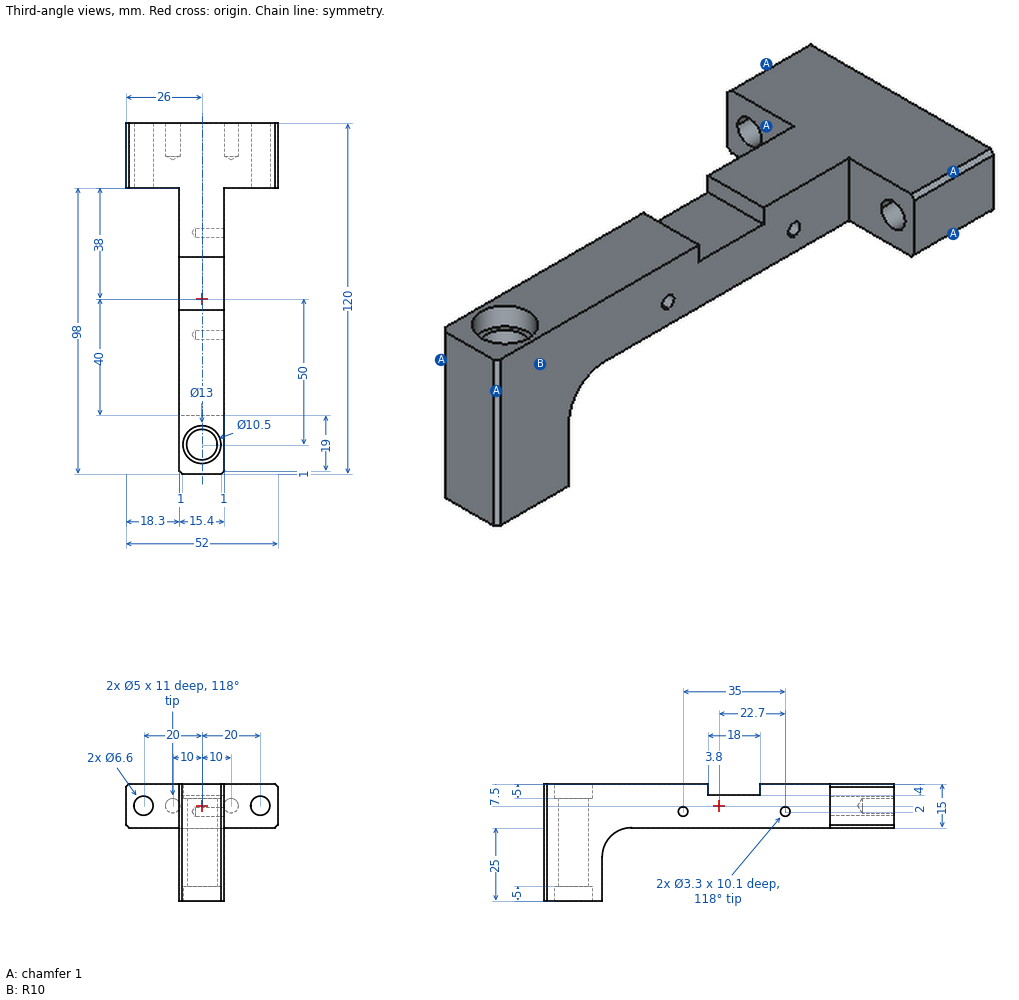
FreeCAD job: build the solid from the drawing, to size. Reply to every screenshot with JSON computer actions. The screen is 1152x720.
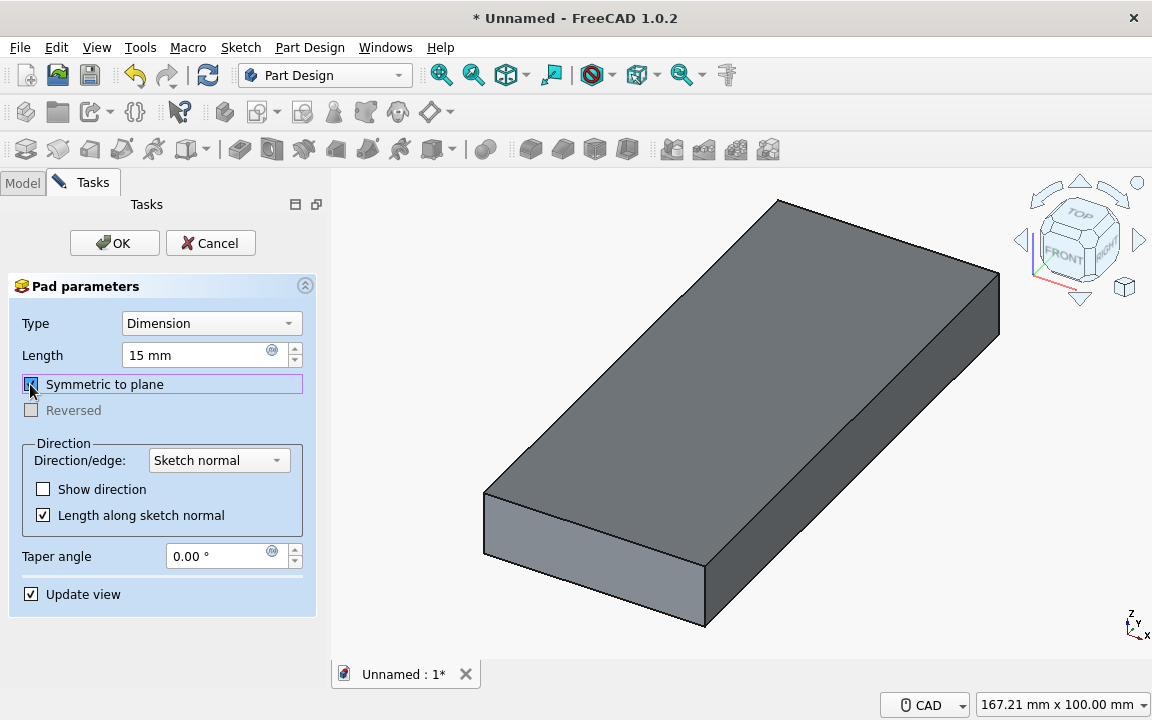
{"action": "left_click", "coordinate": [115, 243]}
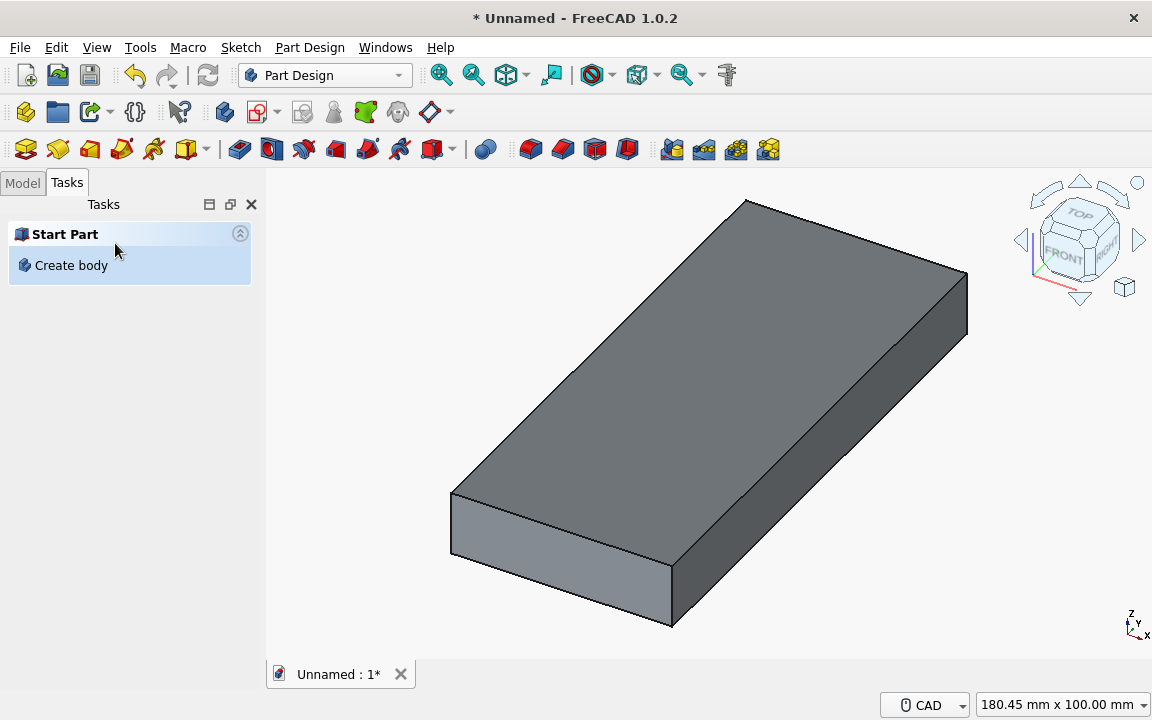
{"action": "left_click", "coordinate": [751, 341]}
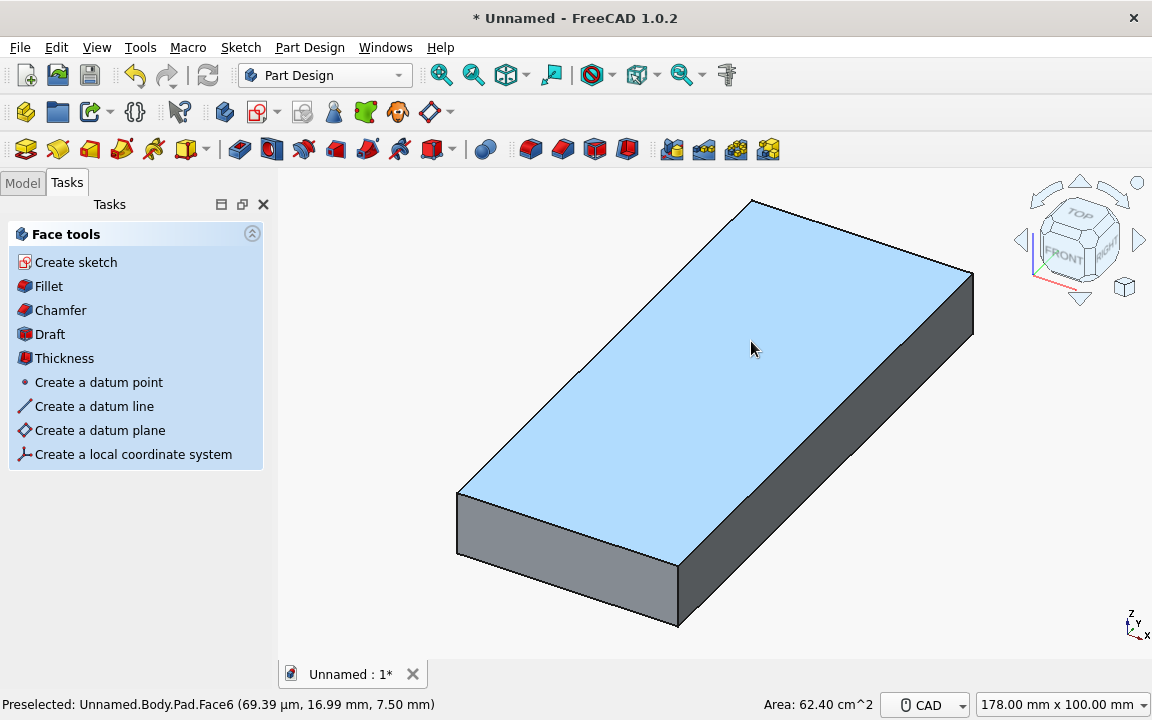
{"action": "left_click", "coordinate": [258, 112]}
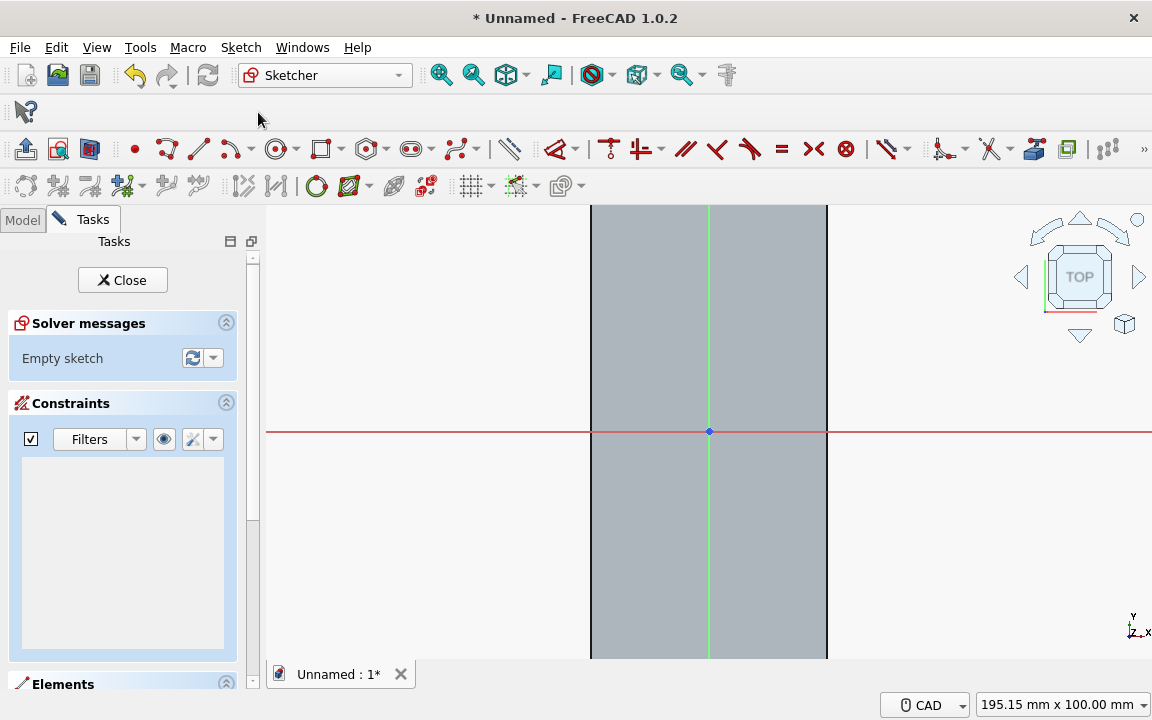
{"action": "scroll", "coordinate": [621, 330], "scroll_direction": "down", "scroll_amount": 2}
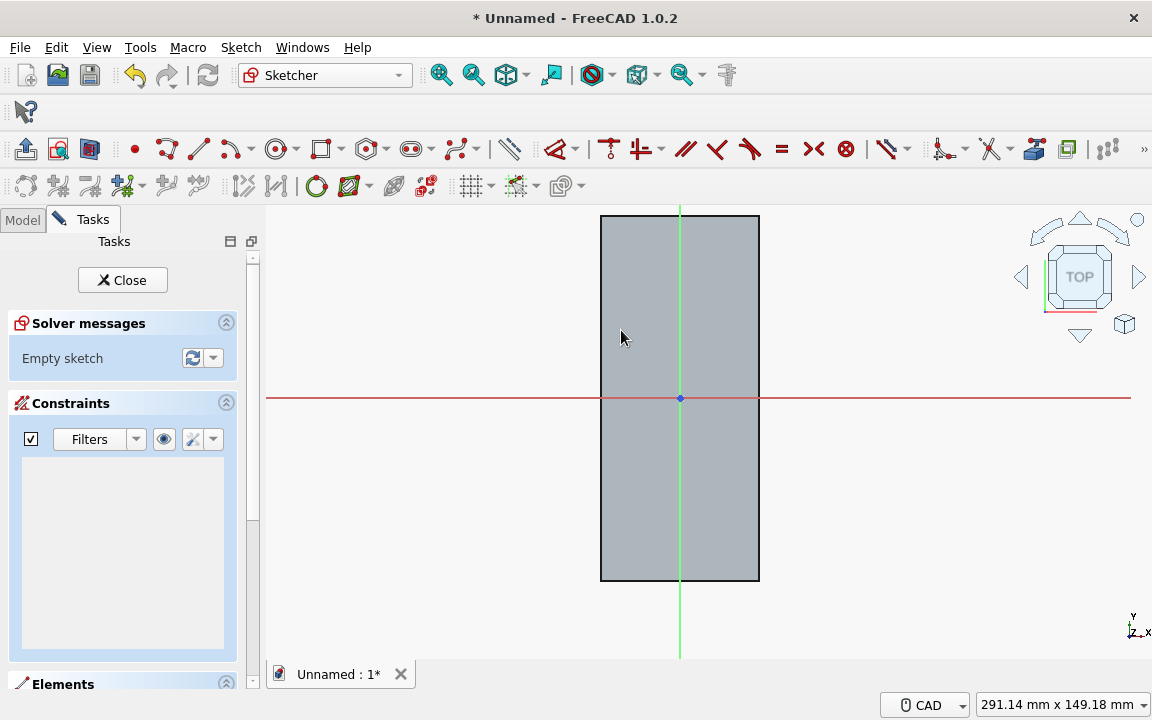
{"action": "left_click", "coordinate": [322, 150]}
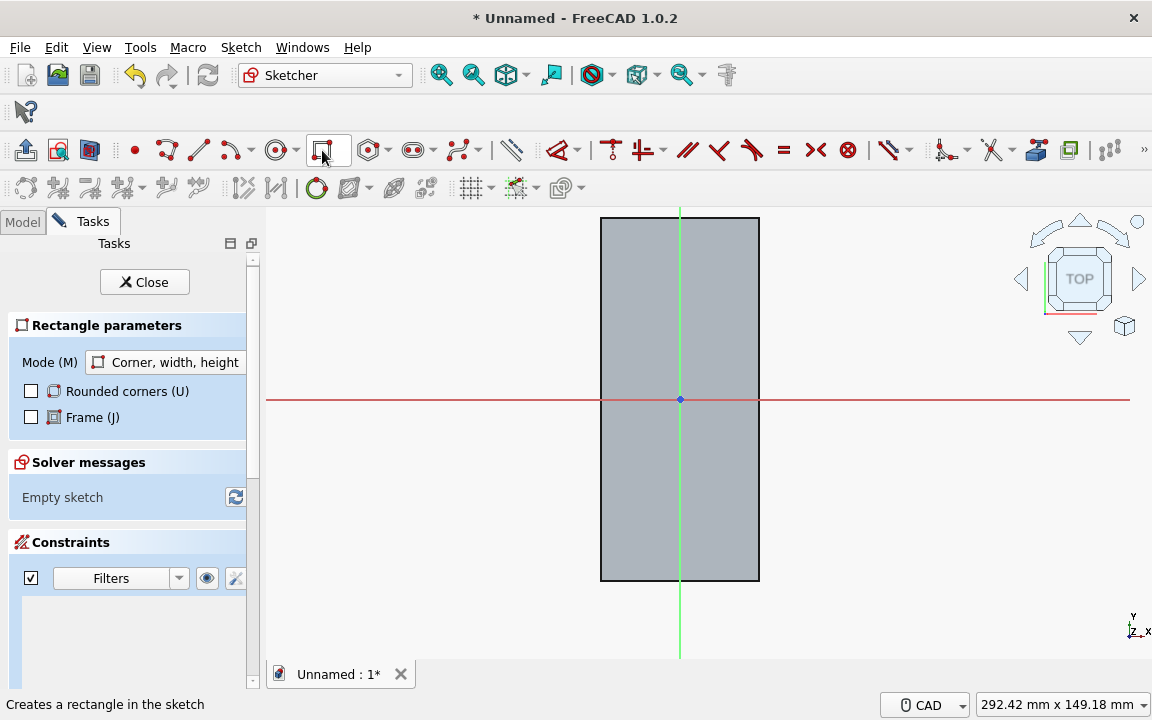
{"action": "left_click", "coordinate": [601, 284]}
{"action": "mouse_move", "coordinate": [657, 581]}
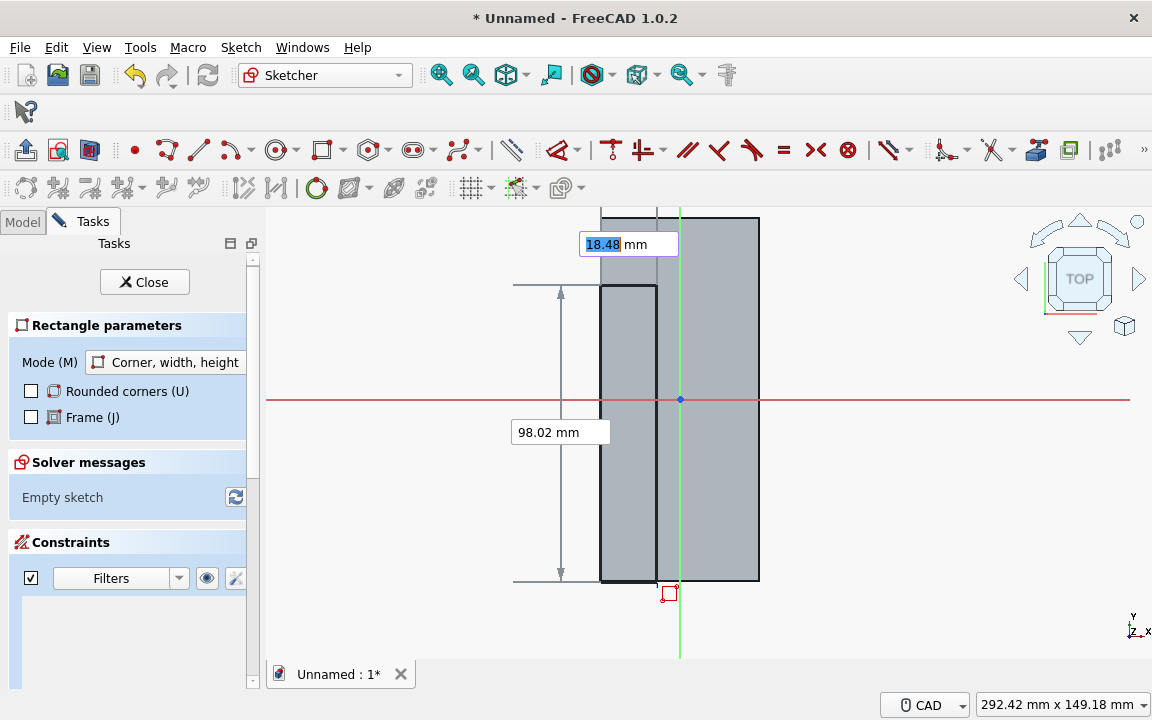
{"action": "type", "text": "18.3"}
{"action": "key", "text": "Tab"}
{"action": "type", "text": "98"}
{"action": "key", "text": "Return"}
{"action": "key", "text": "Escape"}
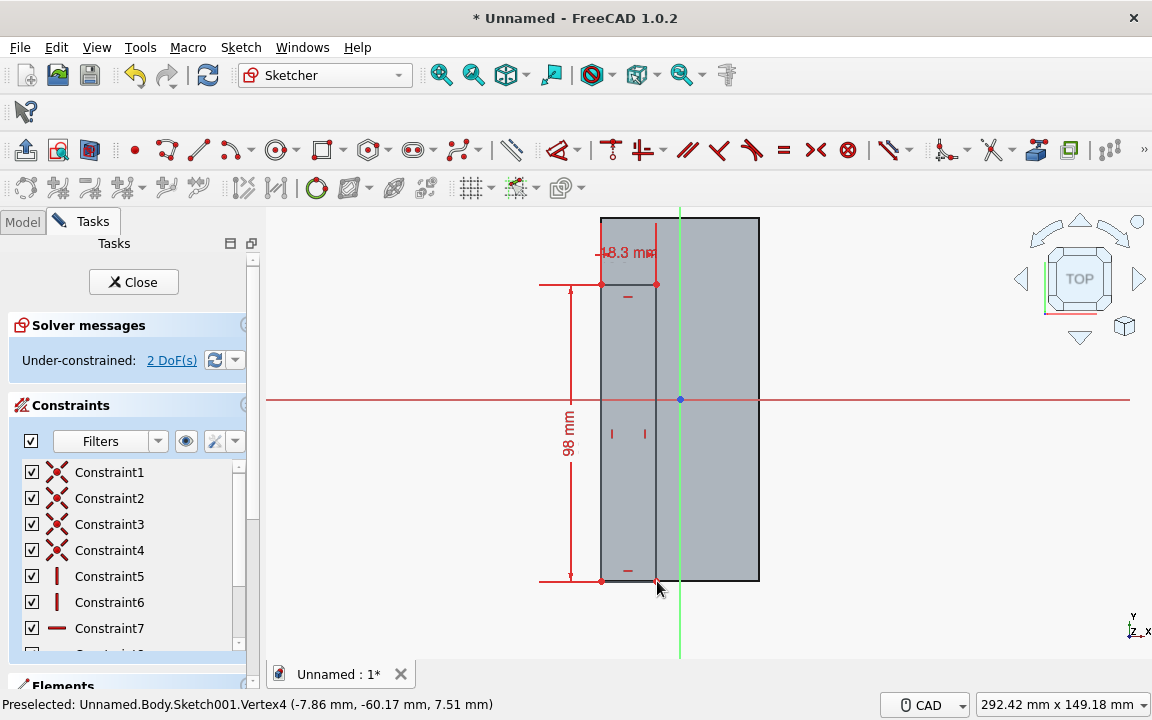
{"action": "left_click", "coordinate": [558, 150]}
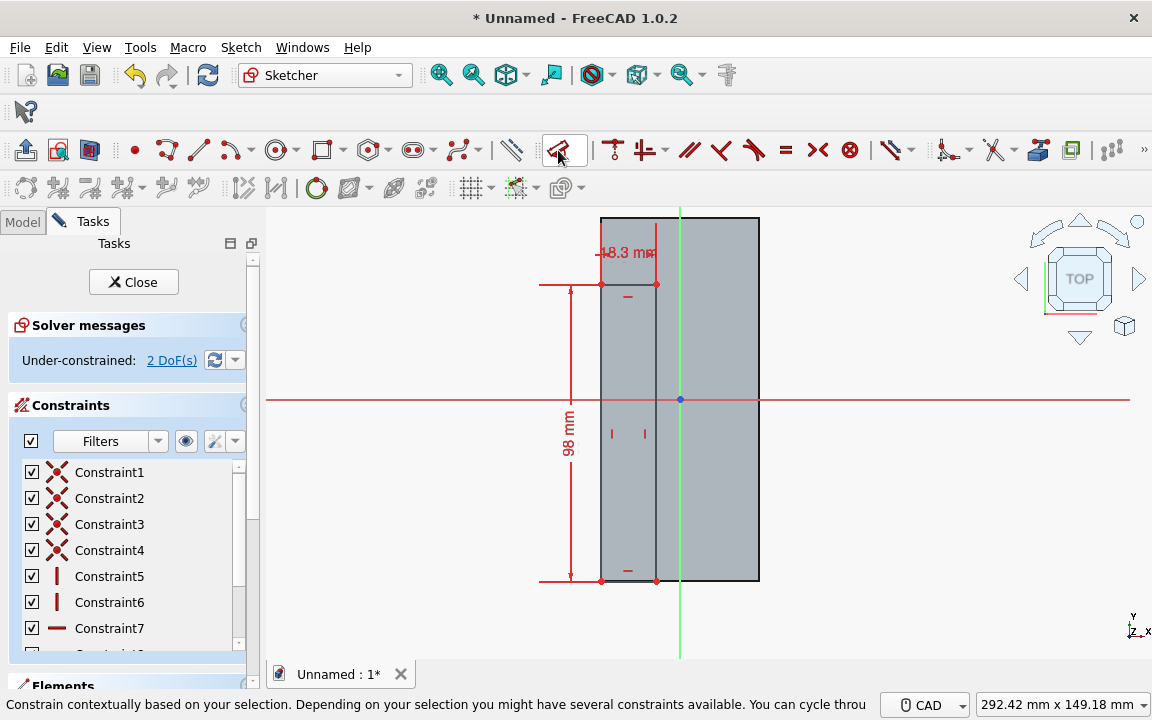
{"action": "left_click", "coordinate": [601, 285]}
{"action": "left_click", "coordinate": [641, 251]}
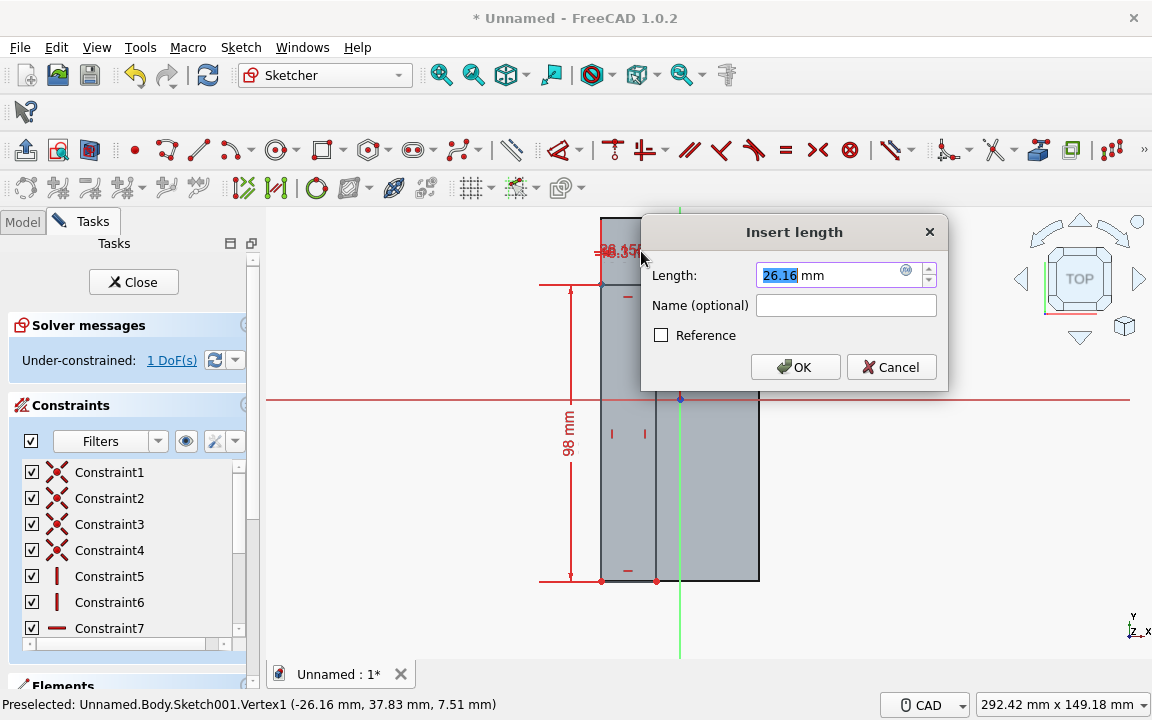
{"action": "type", "text": "26"}
{"action": "key", "text": "Return"}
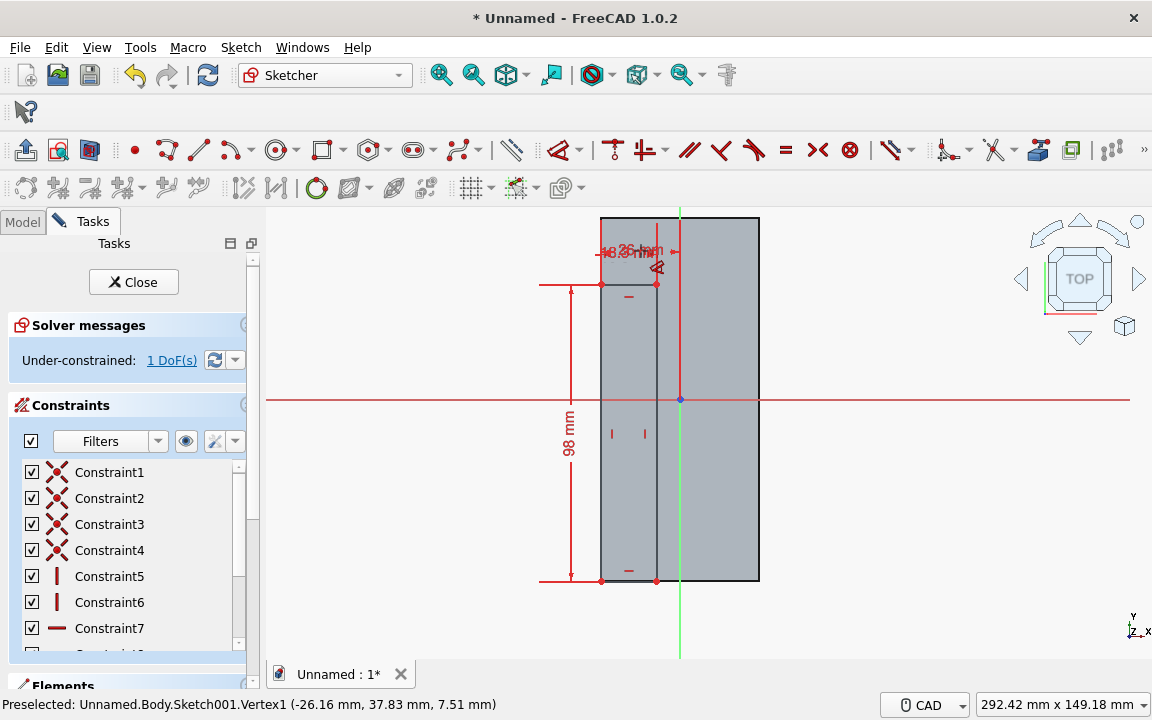
{"action": "left_click", "coordinate": [601, 285]}
{"action": "left_click", "coordinate": [714, 342]}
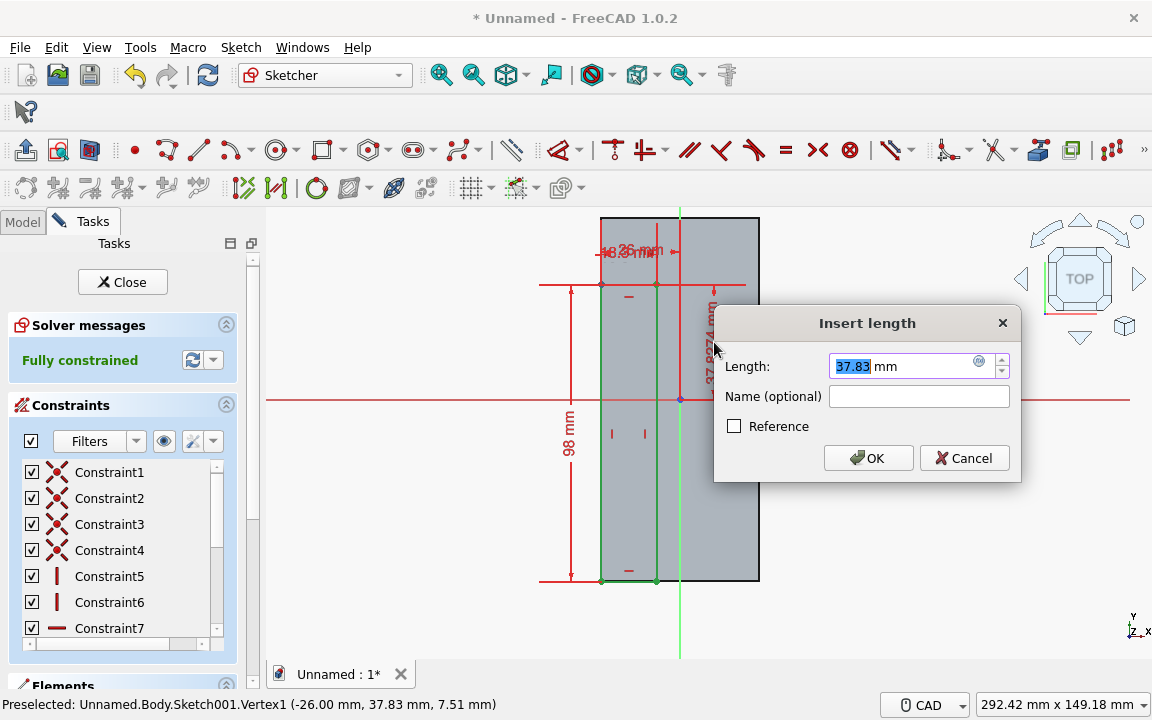
{"action": "type", "text": "38"}
{"action": "key", "text": "Return"}
{"action": "key", "text": "Escape"}